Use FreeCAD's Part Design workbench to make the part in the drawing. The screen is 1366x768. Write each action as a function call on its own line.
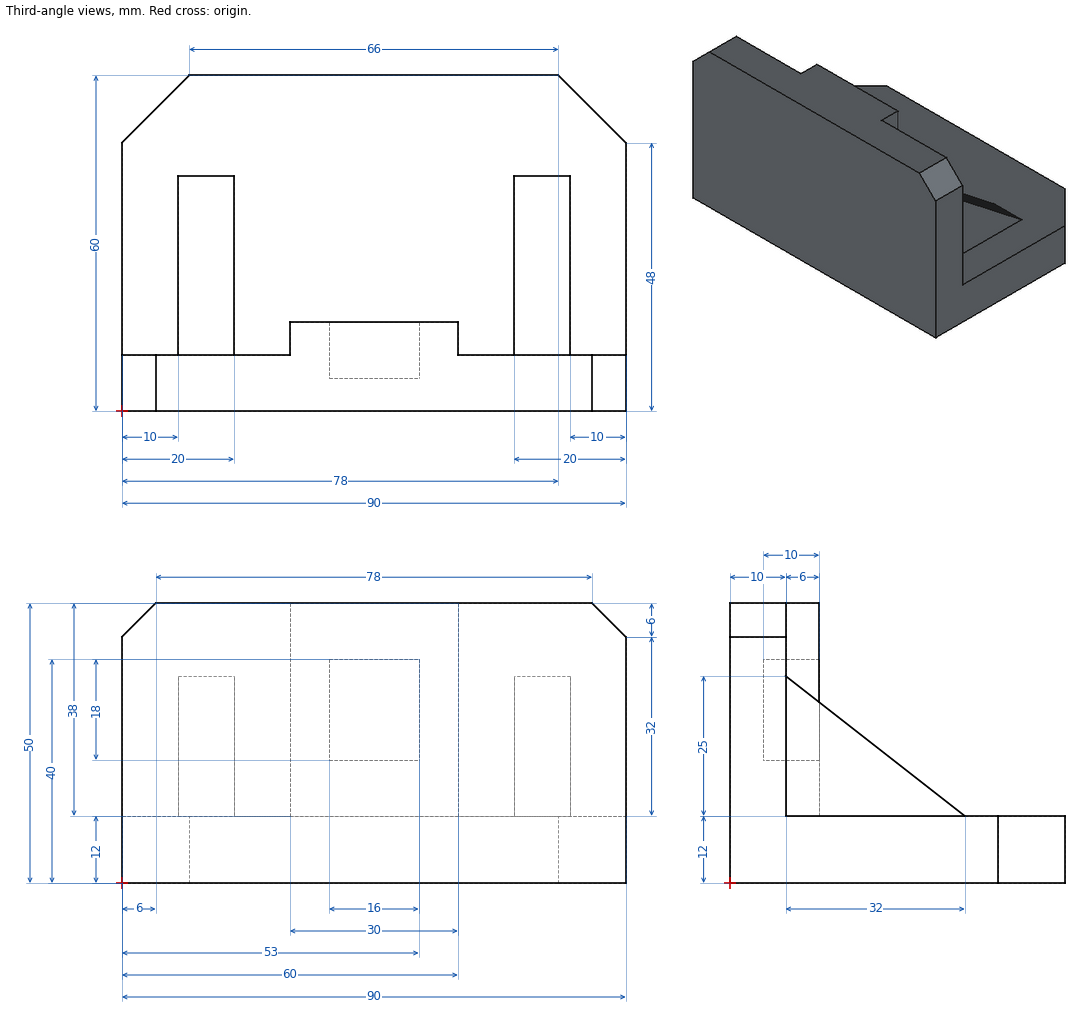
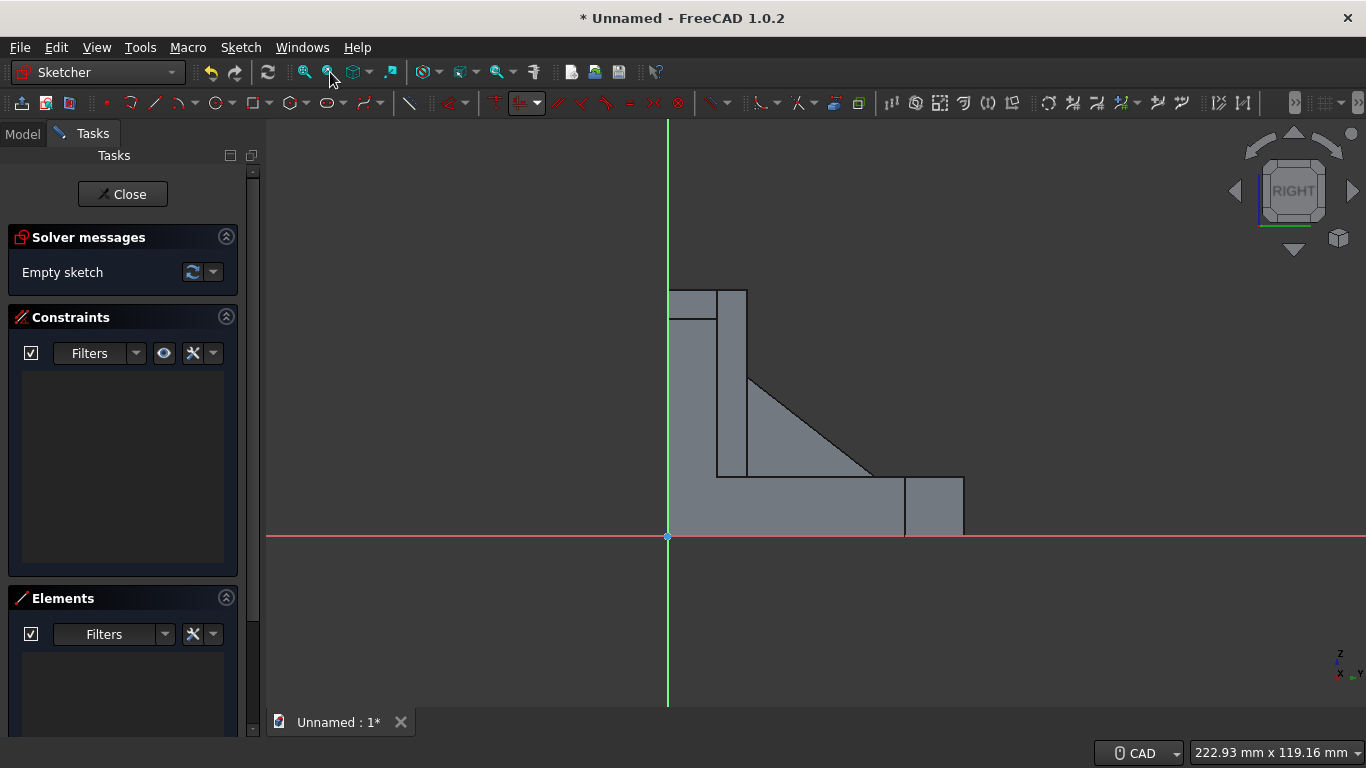
scroll(791, 471, up, 4)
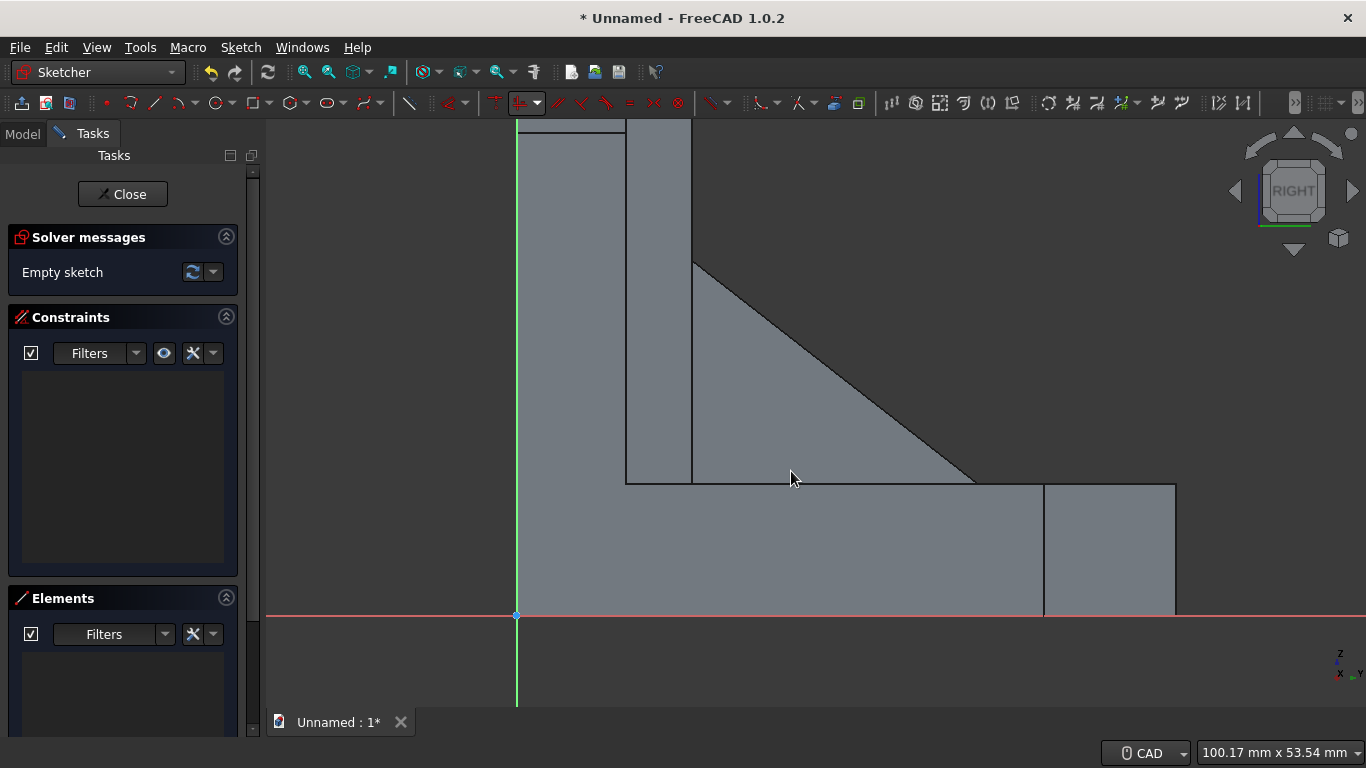
click(132, 104)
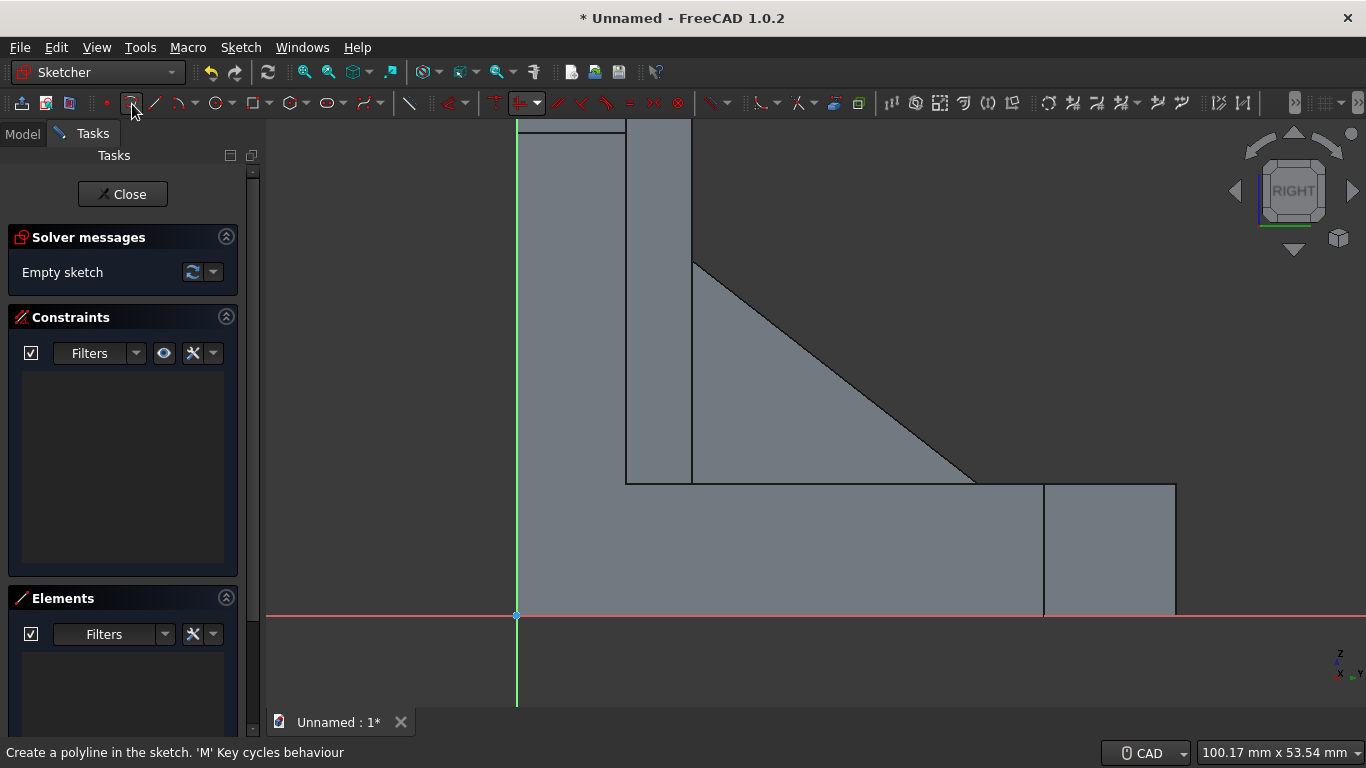
click(626, 484)
click(978, 484)
click(626, 209)
click(626, 485)
key(Escape)
key(Escape)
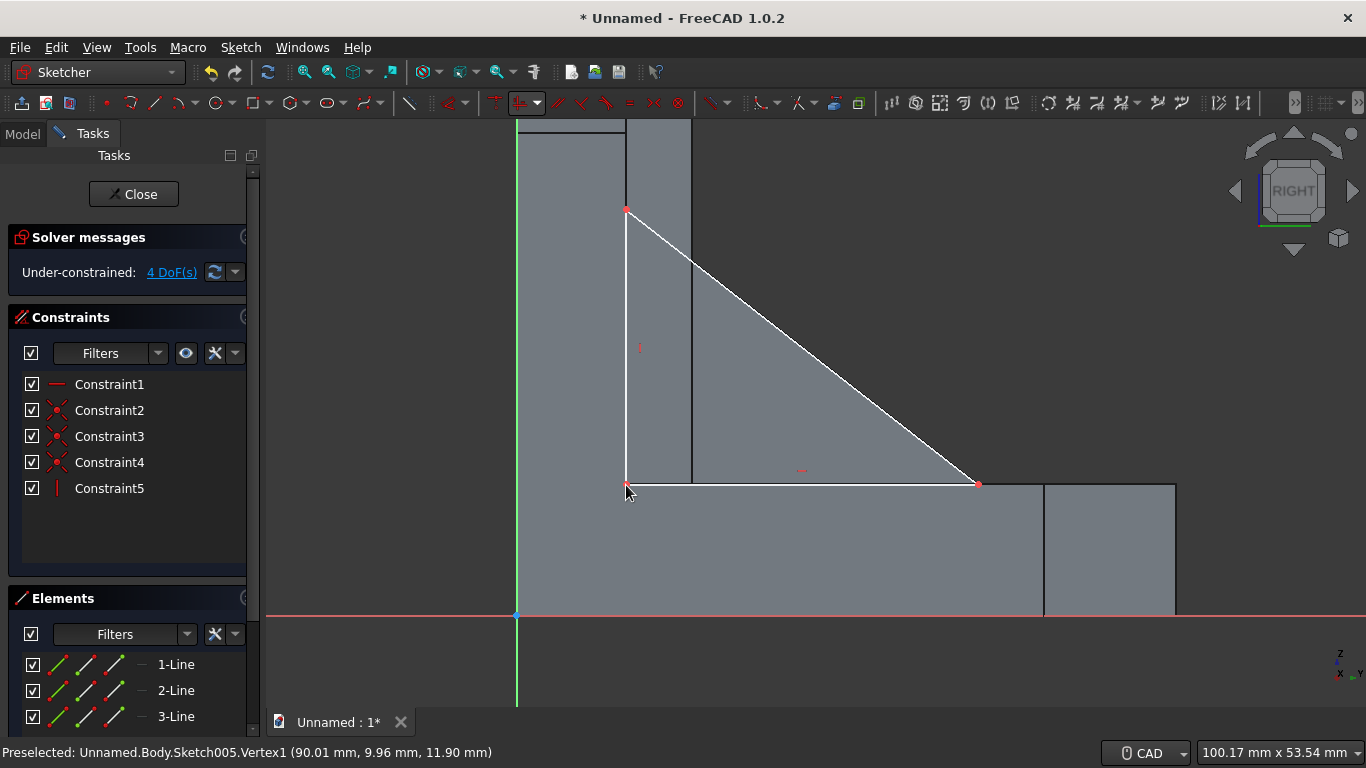
click(448, 104)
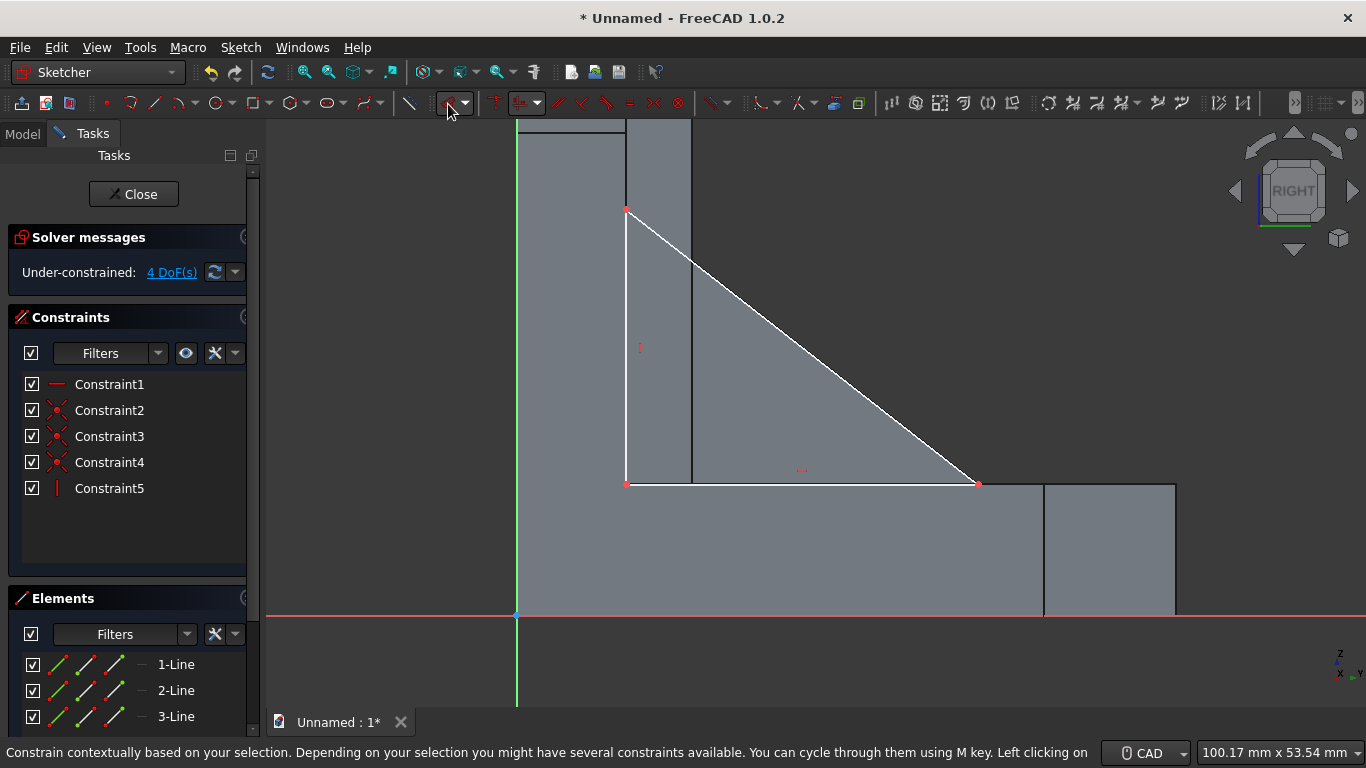
click(732, 485)
click(802, 519)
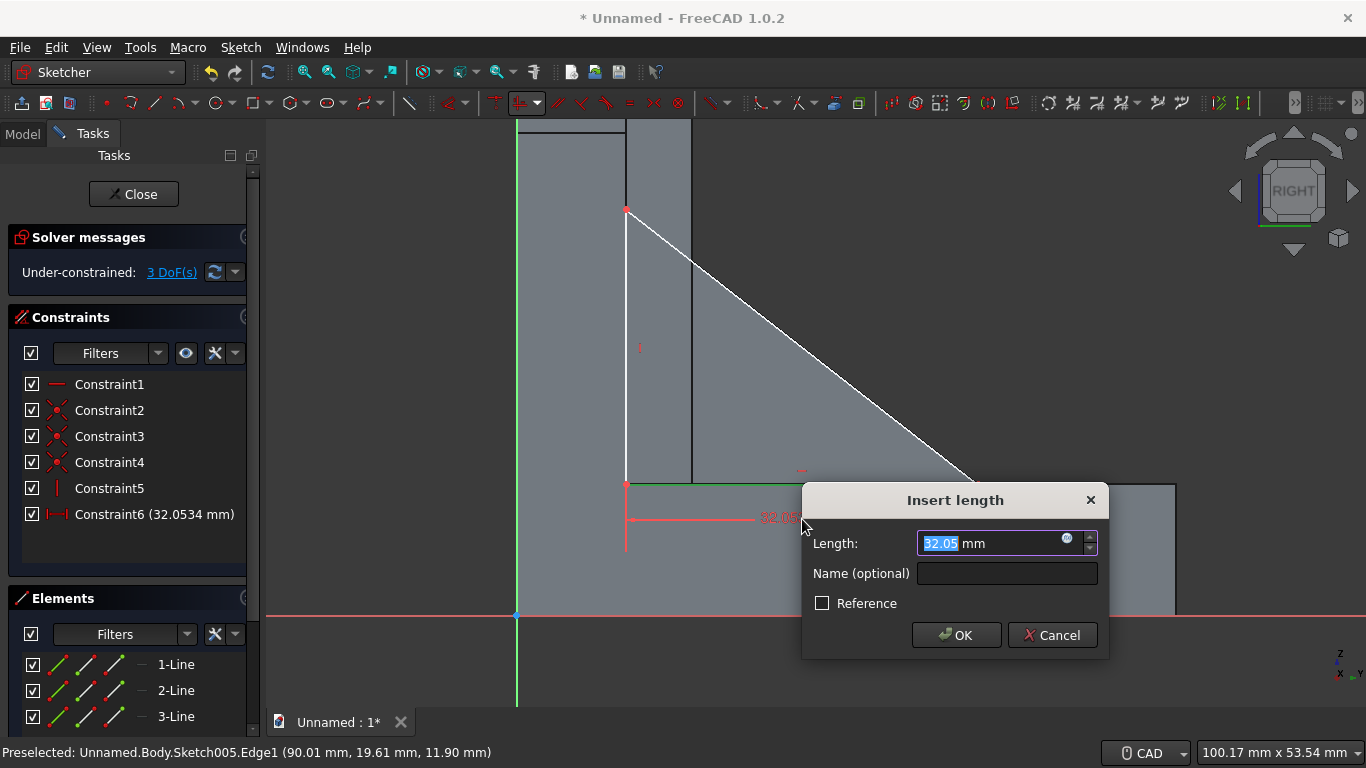
text(32)
key(Return)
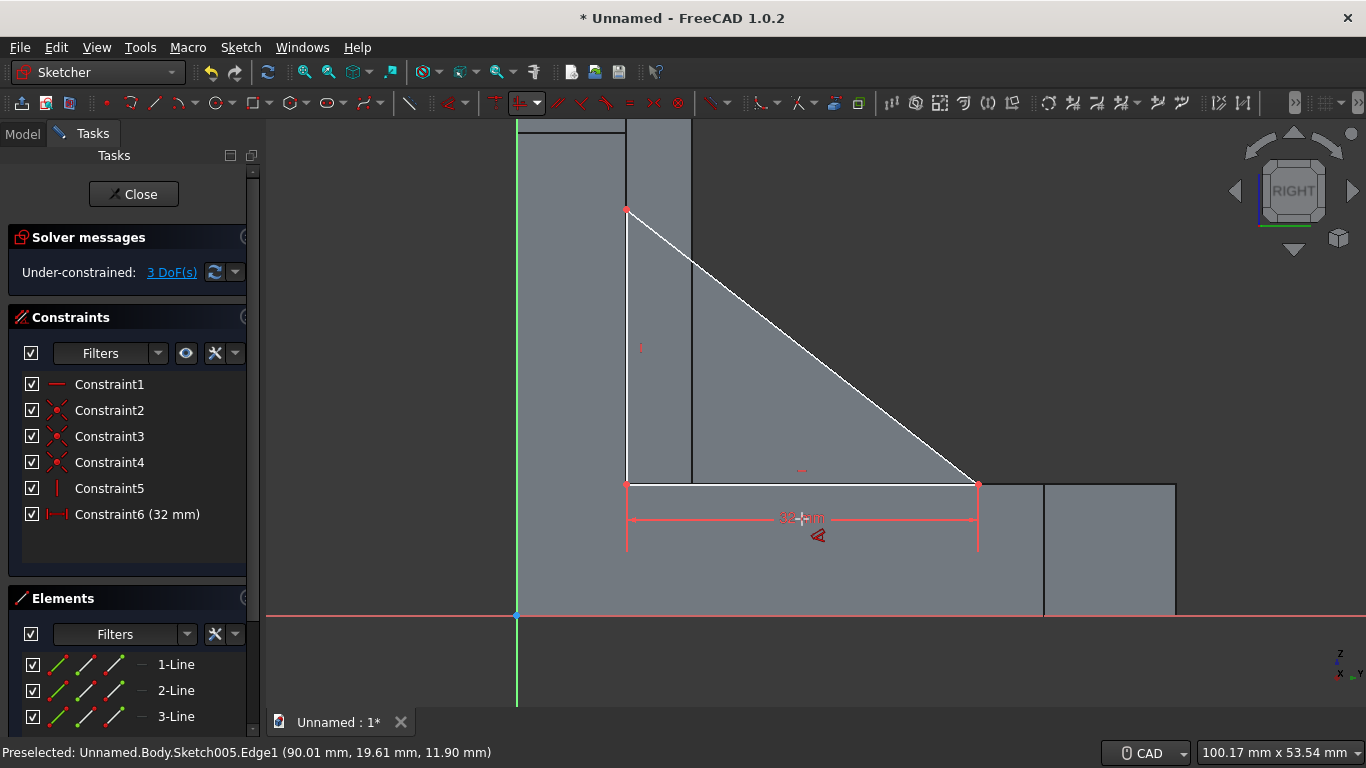
click(627, 292)
click(593, 347)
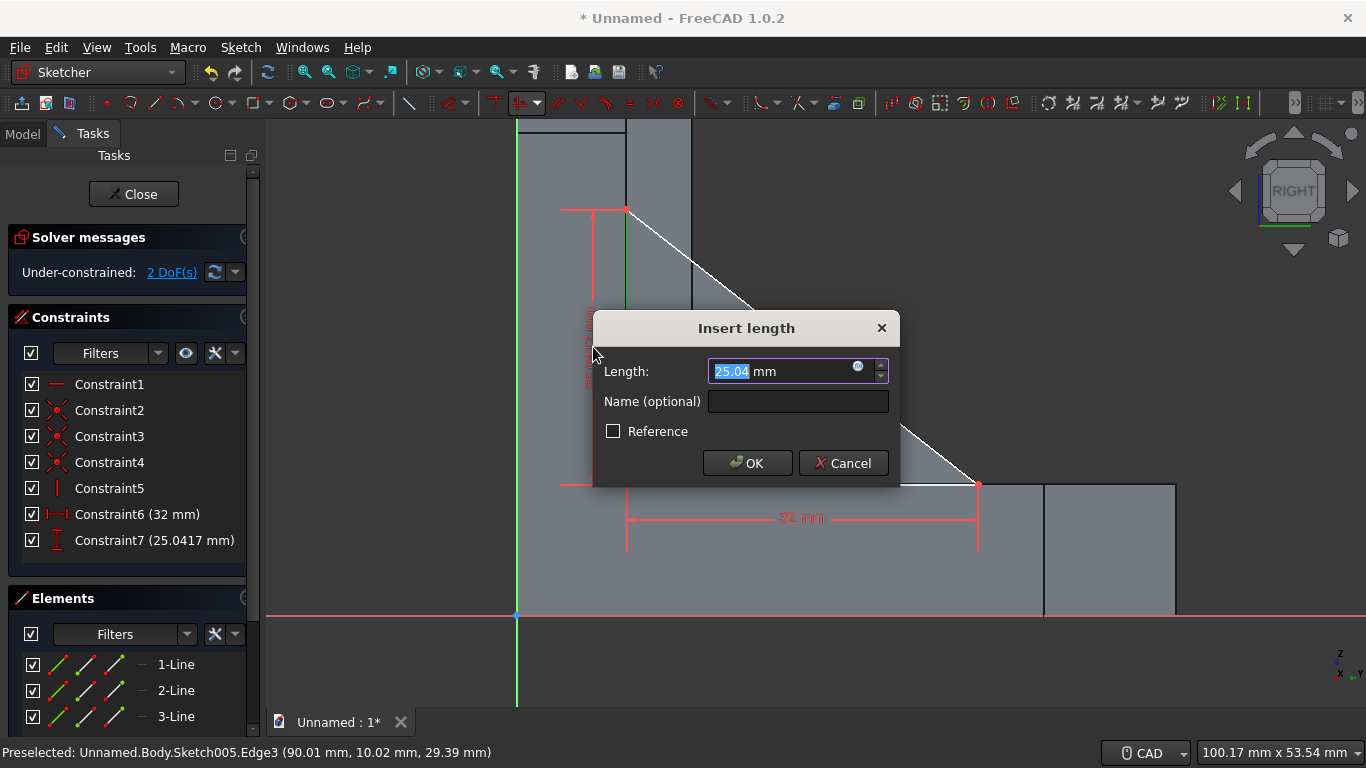
text(25)
key(Return)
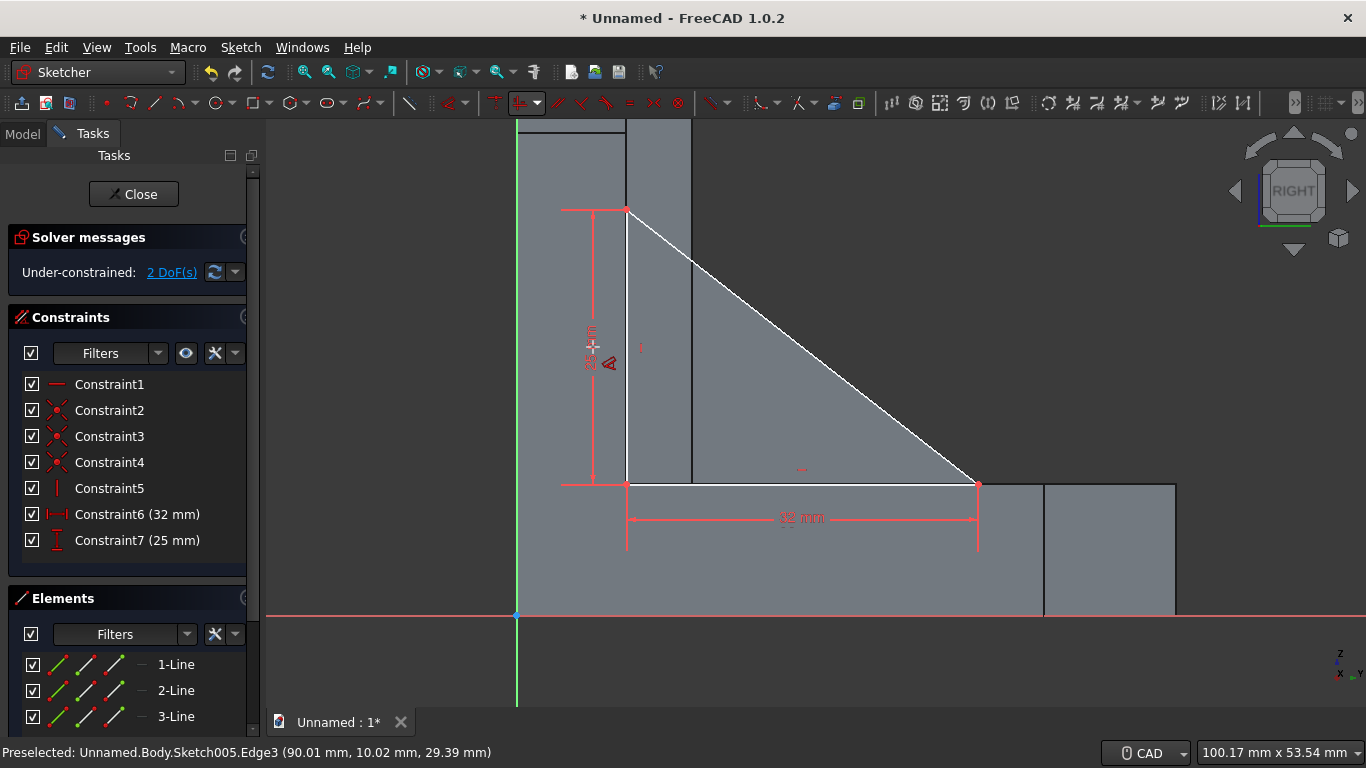
click(627, 485)
click(572, 650)